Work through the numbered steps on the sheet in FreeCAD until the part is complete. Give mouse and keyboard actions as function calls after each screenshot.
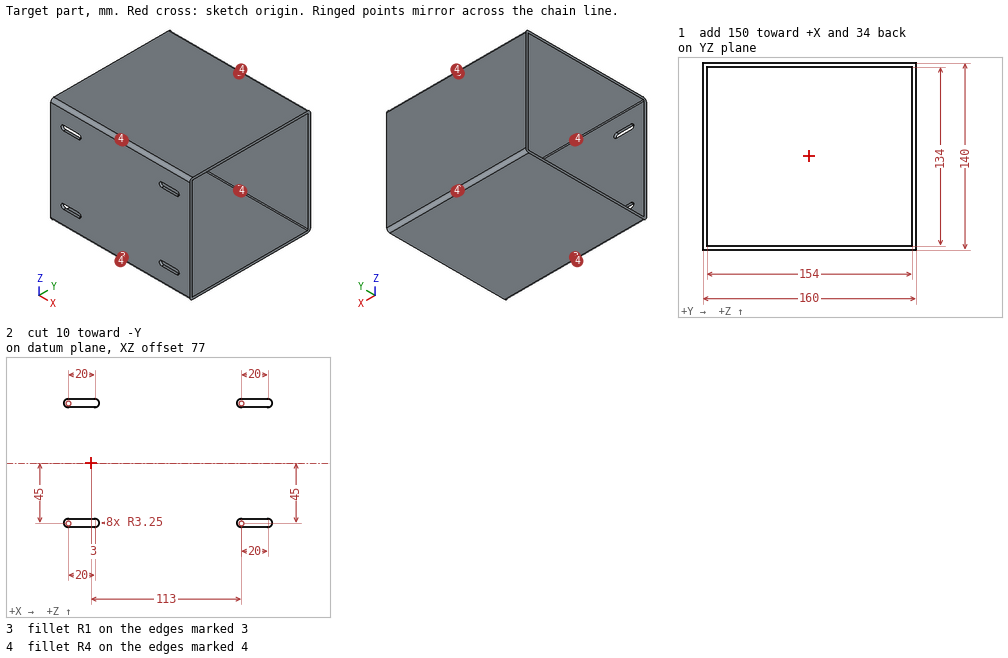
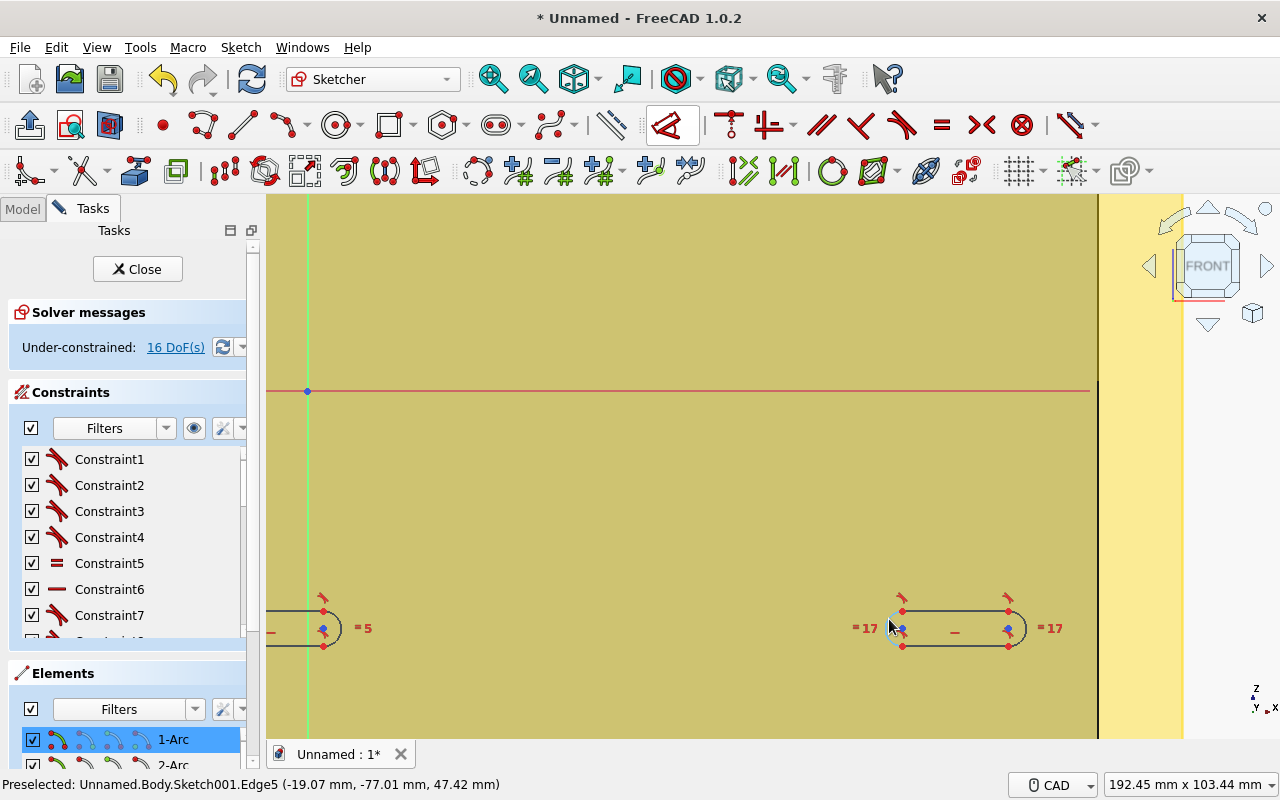
click(889, 619)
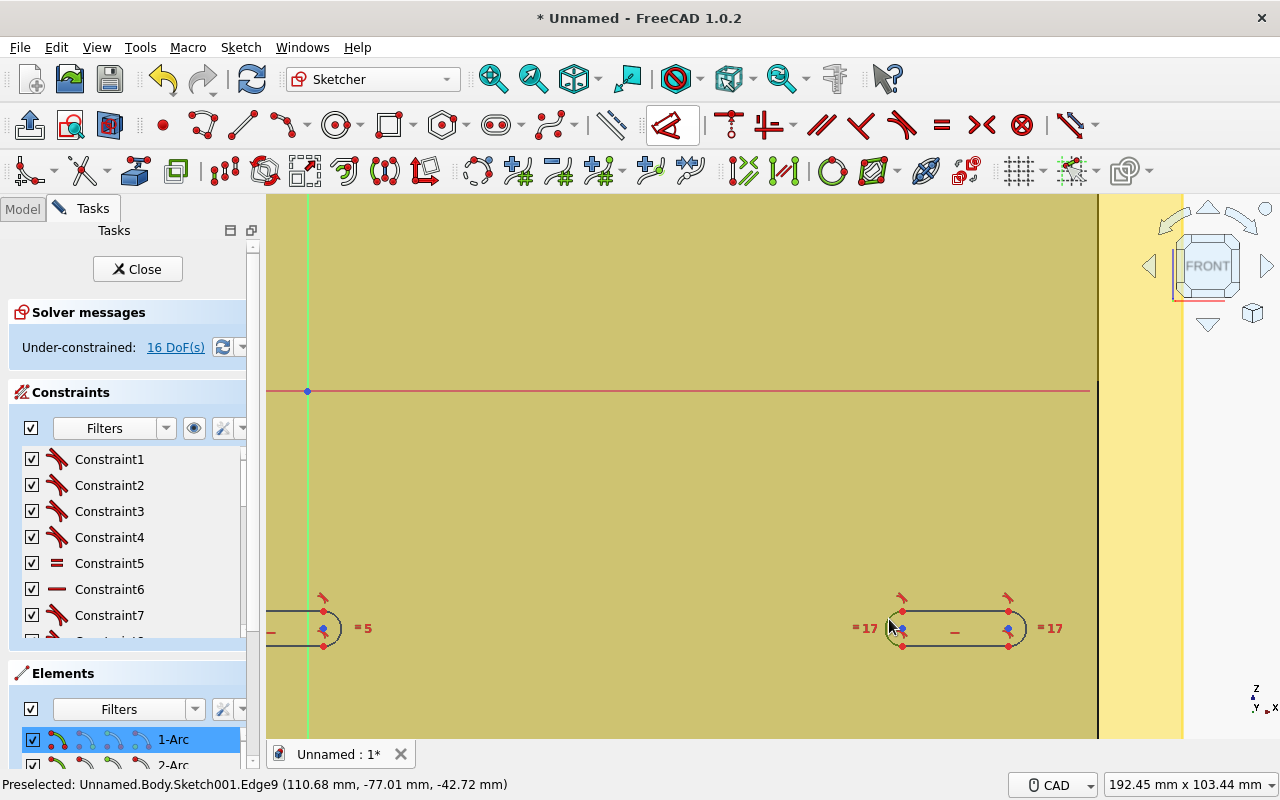
scroll(890, 620, down, 2)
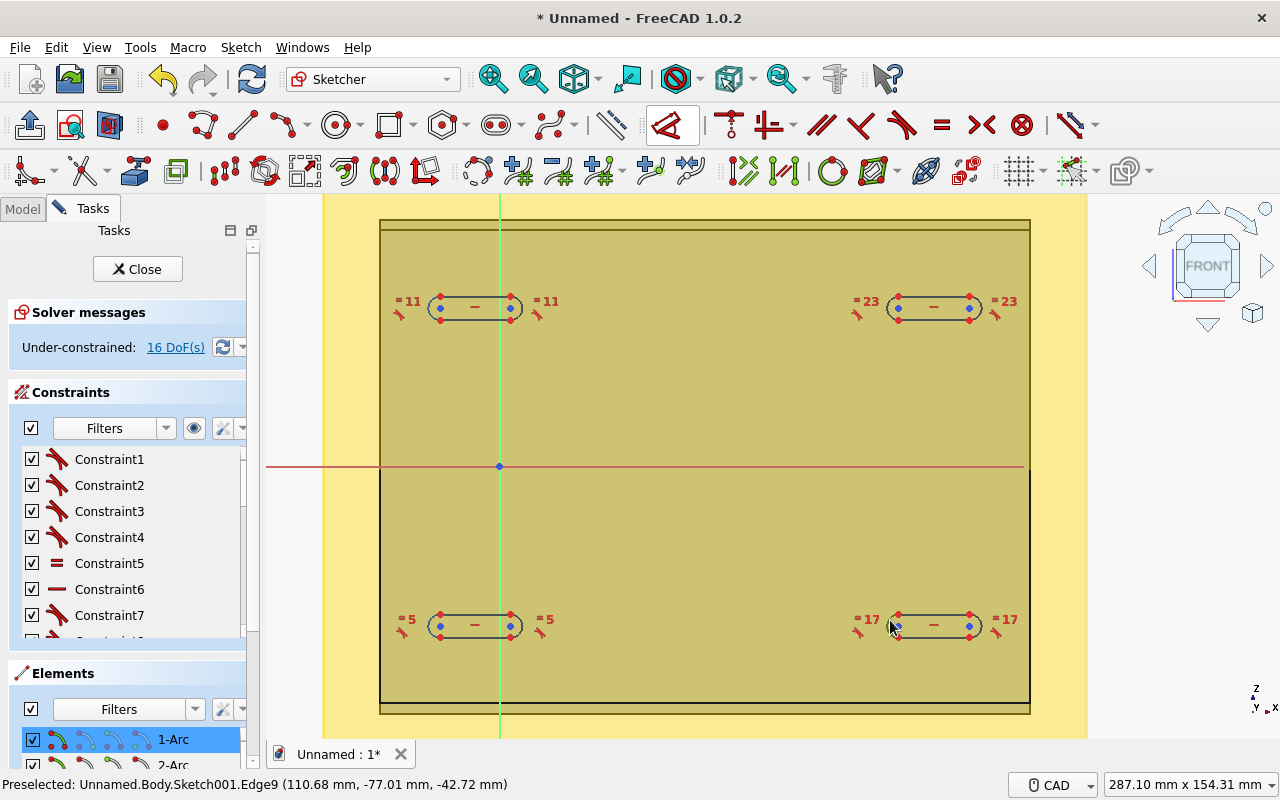
scroll(889, 301, up, 2)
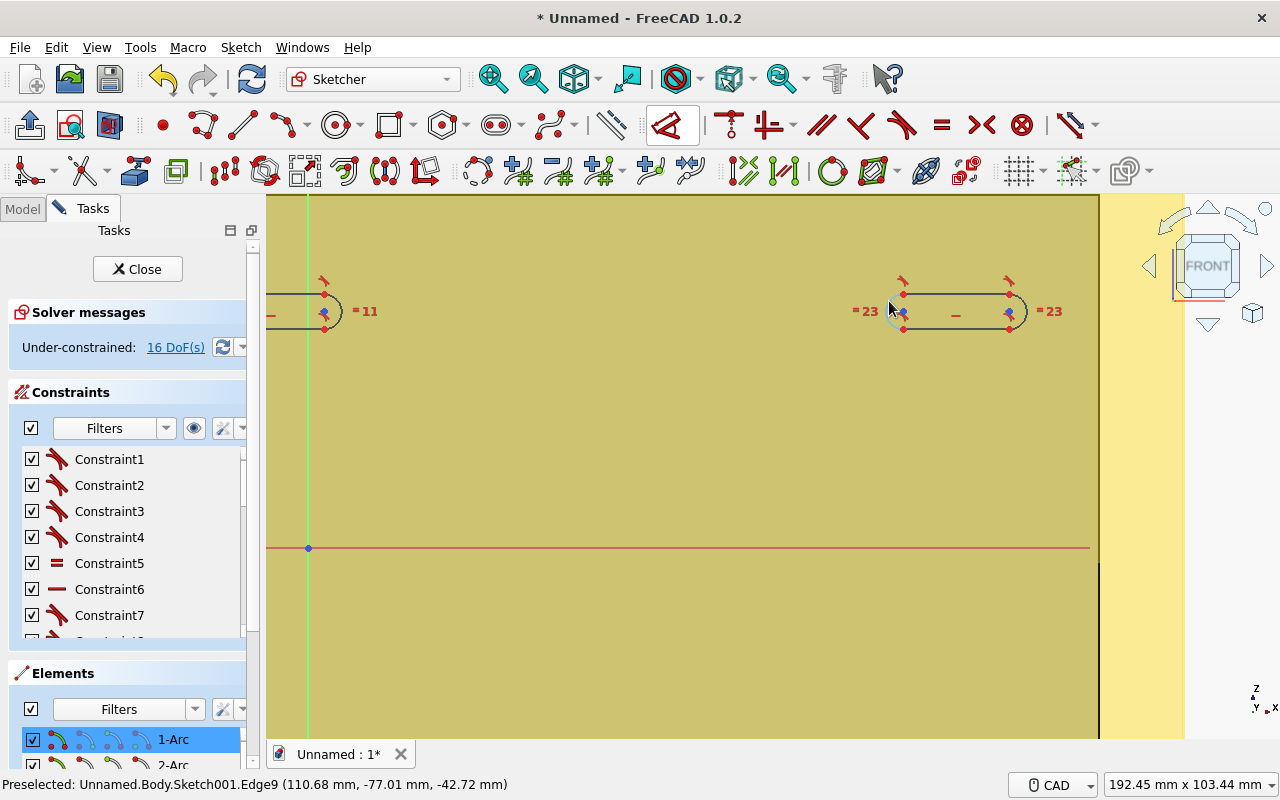
click(889, 302)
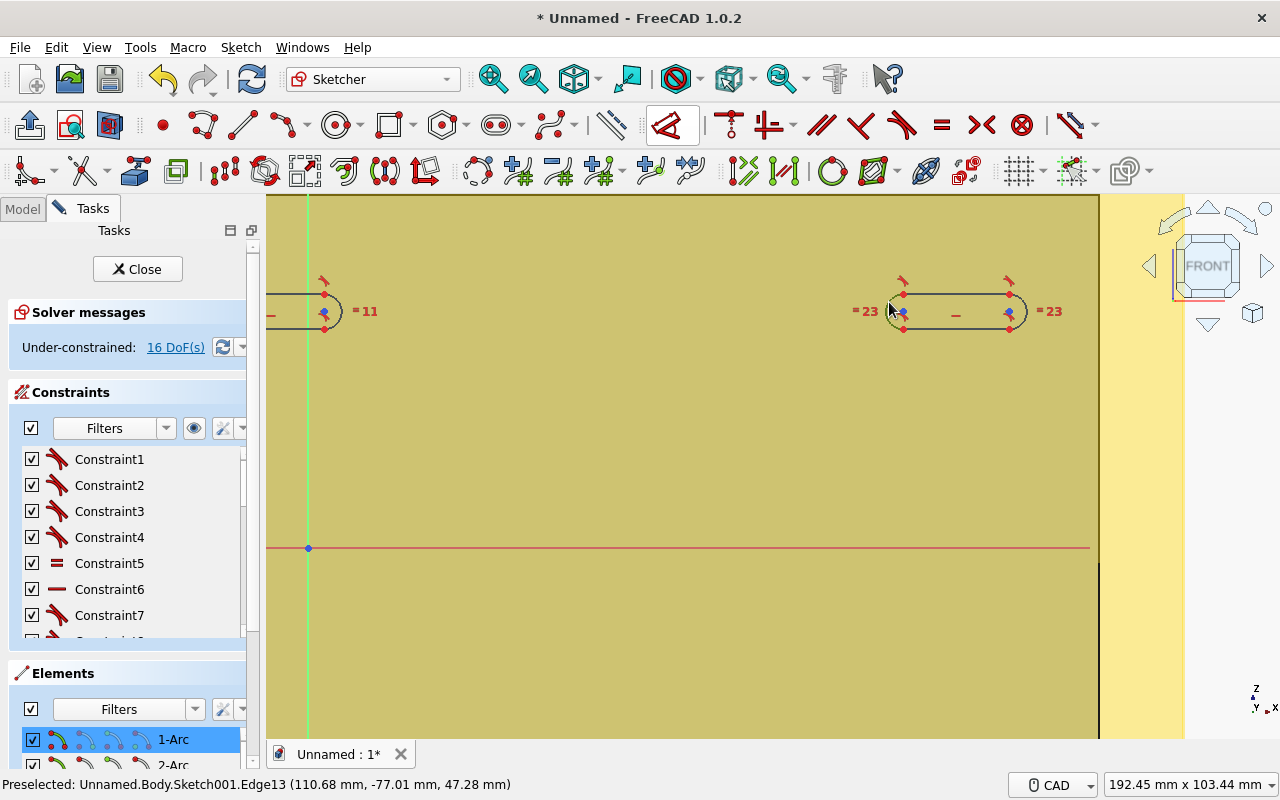
key(e)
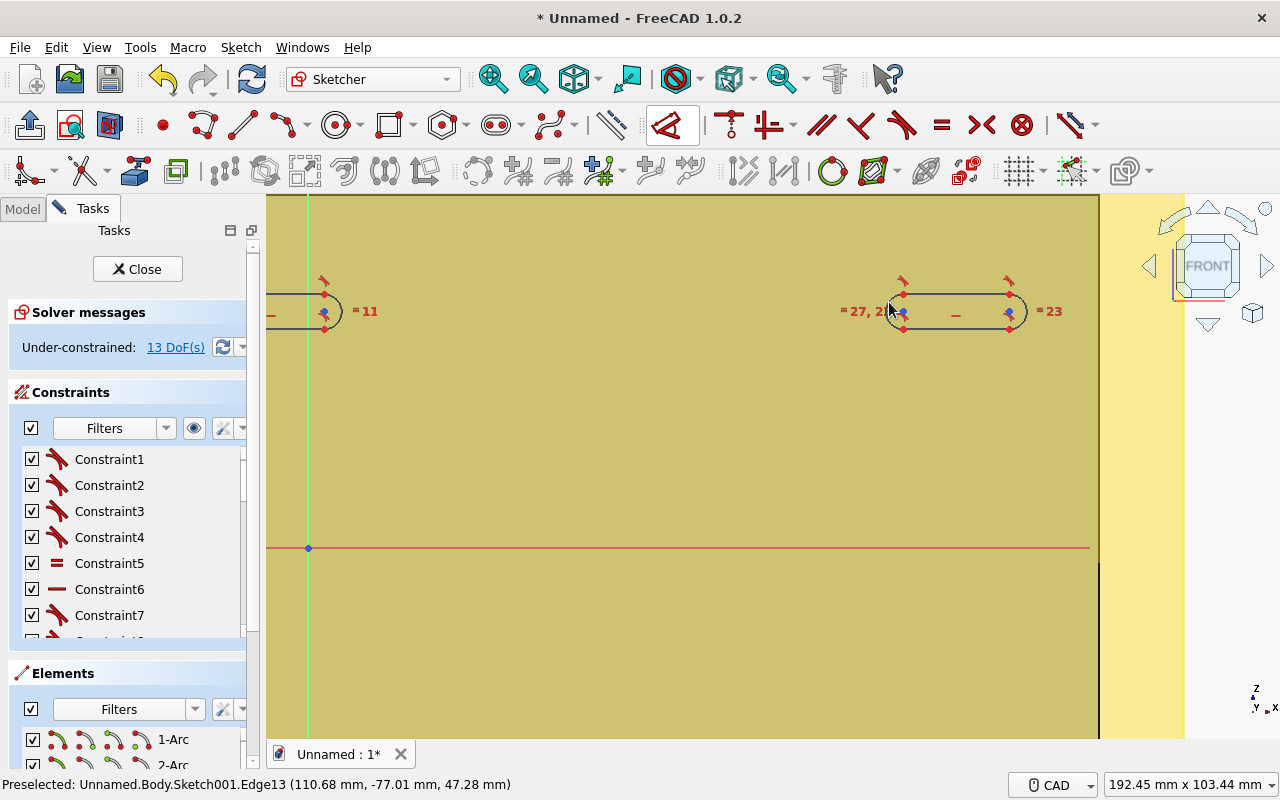
scroll(889, 300, down, 2)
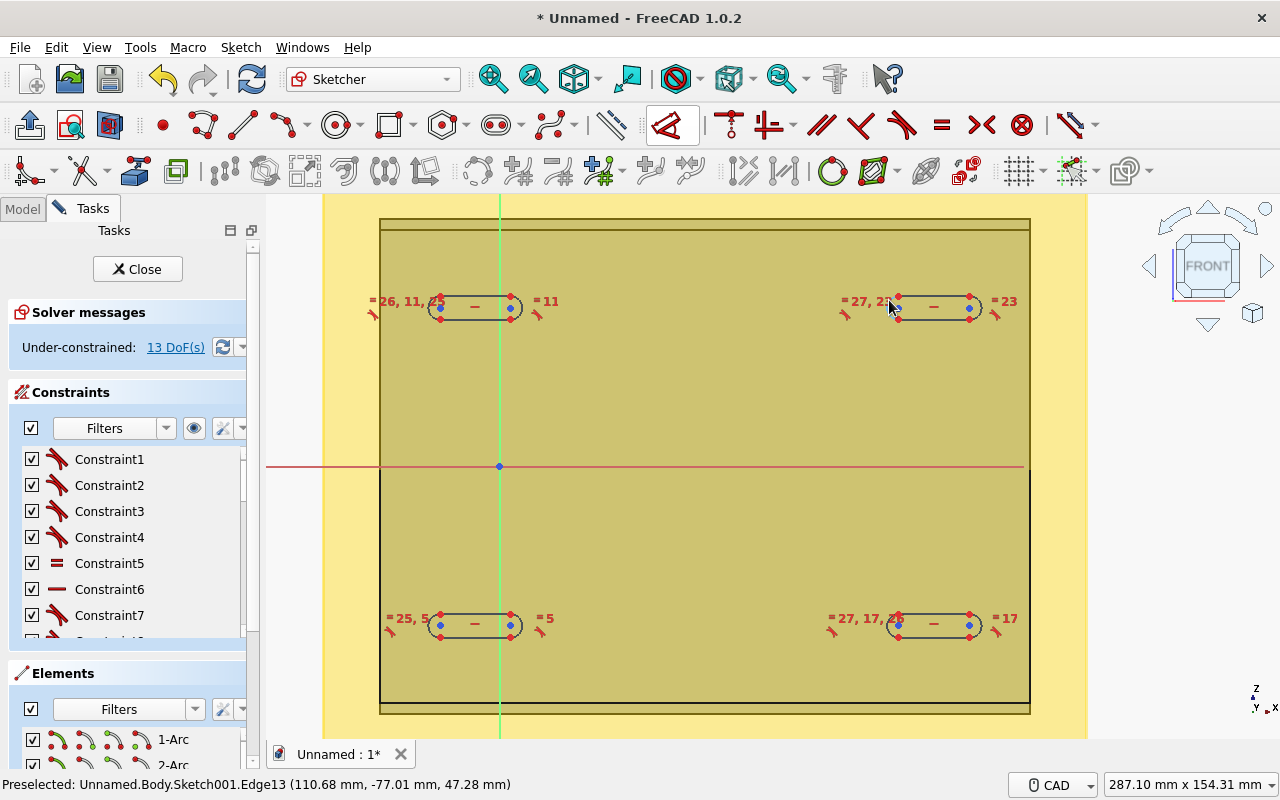
click(440, 626)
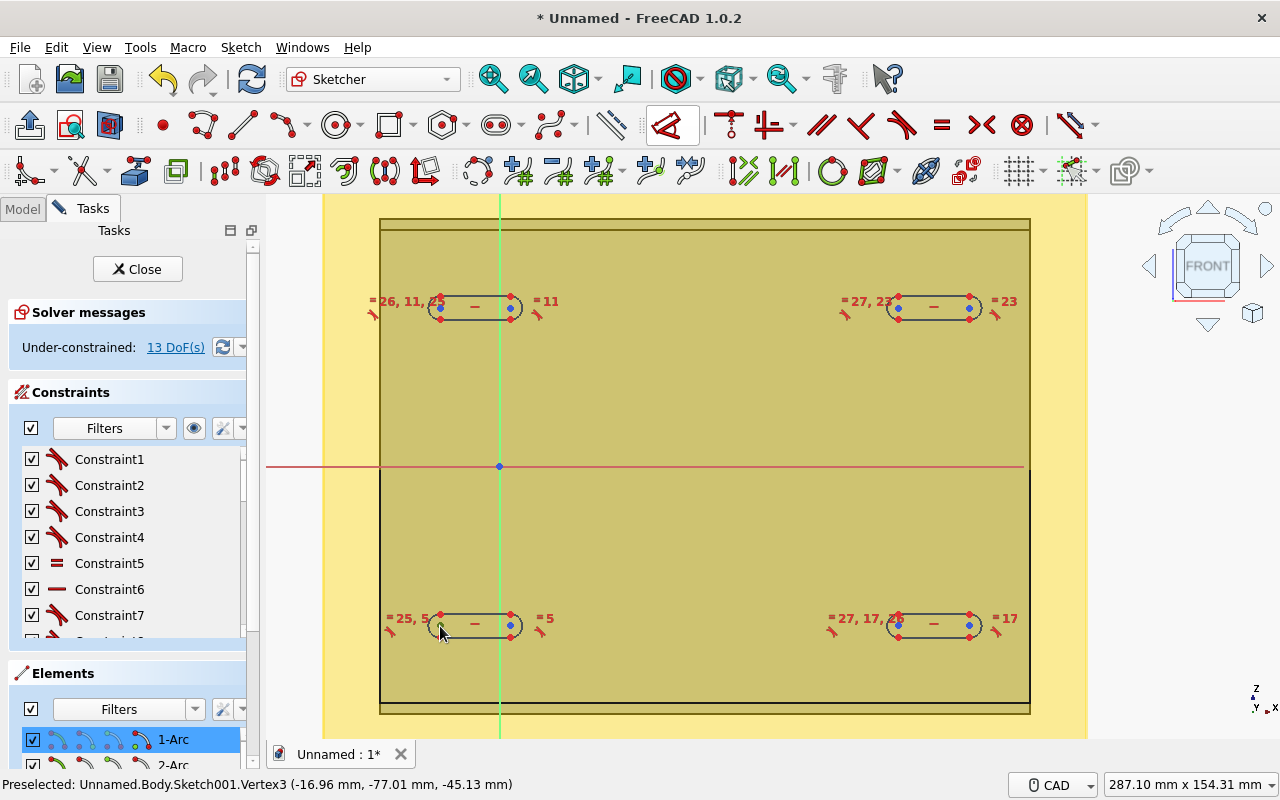
click(440, 308)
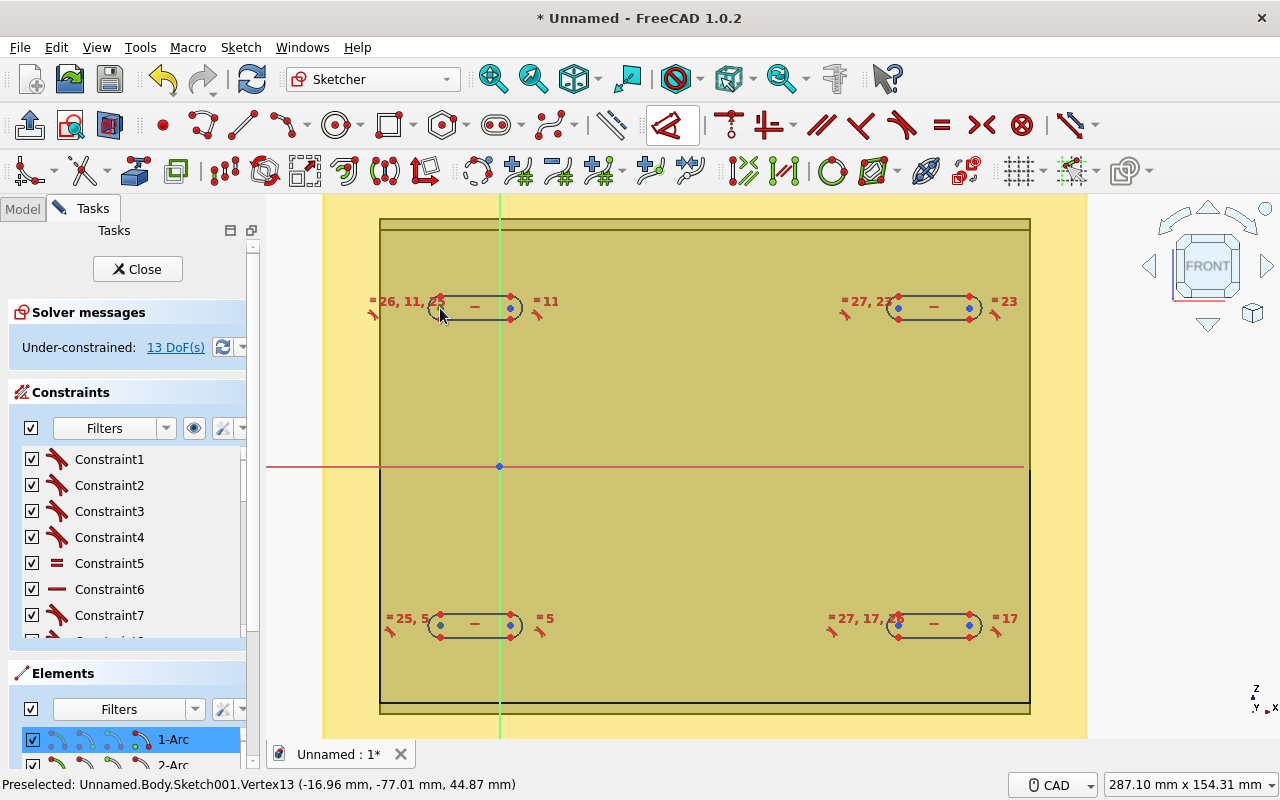
click(353, 466)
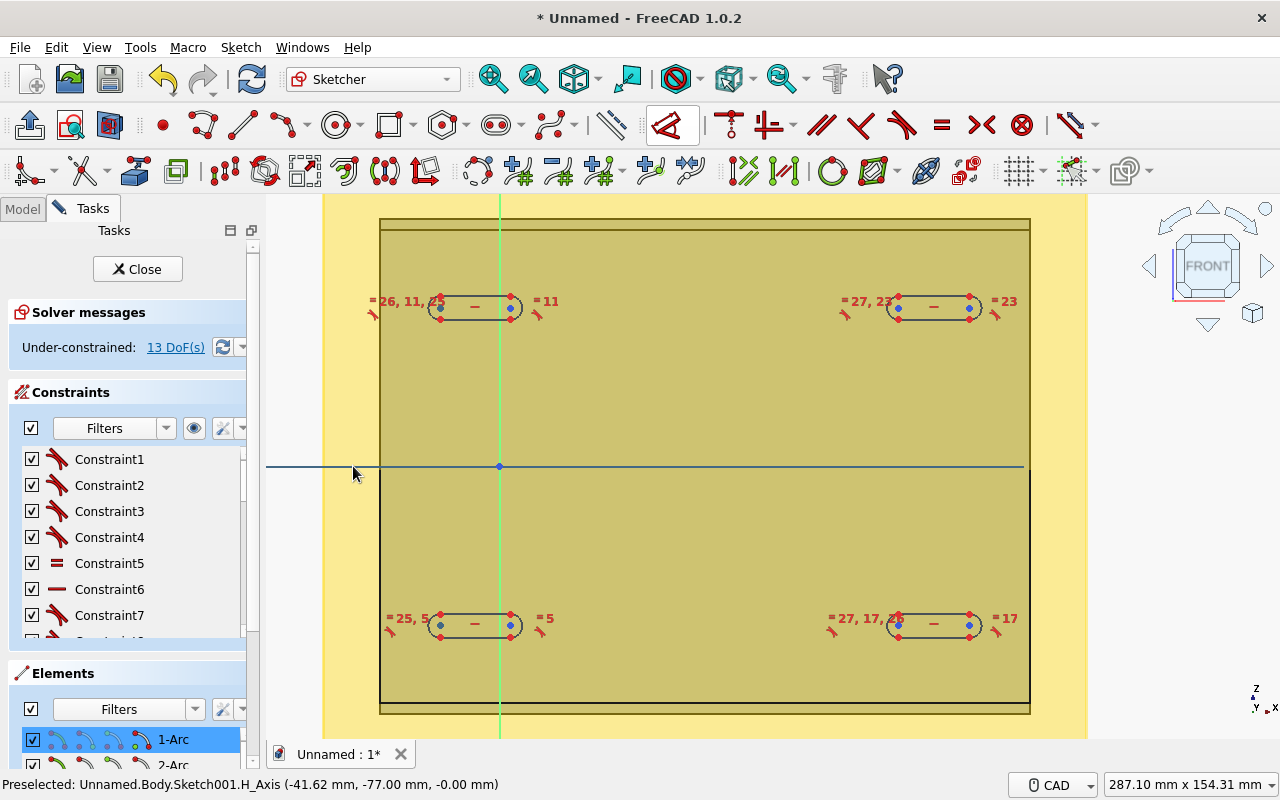
click(982, 126)